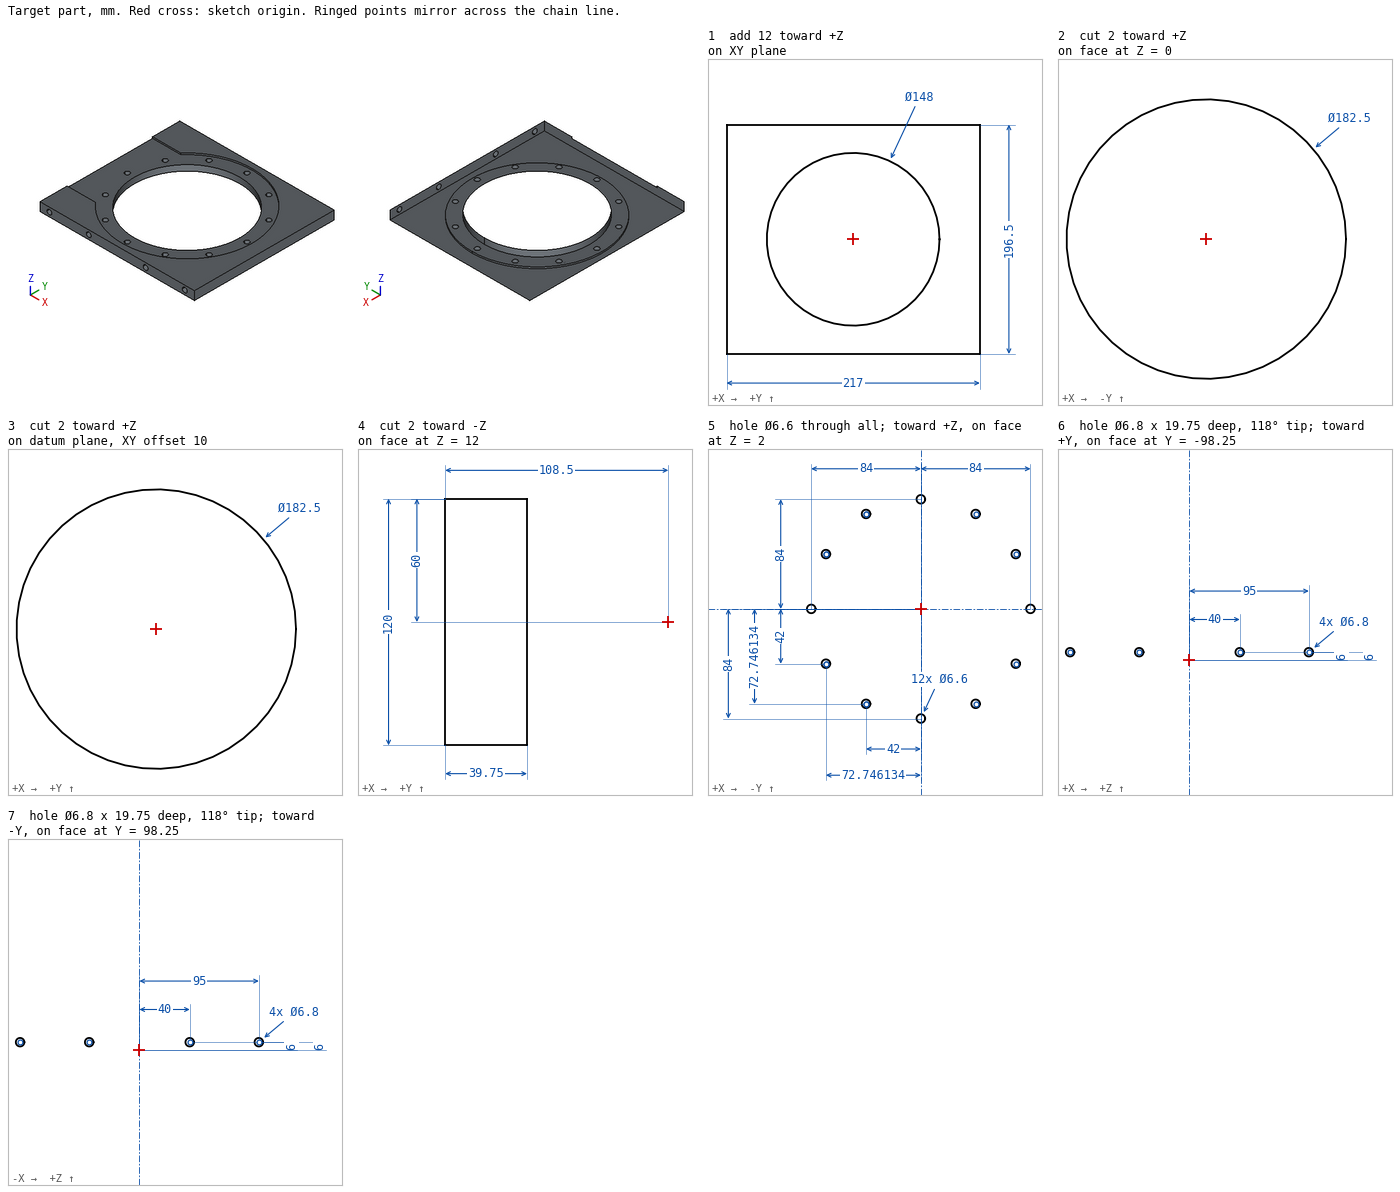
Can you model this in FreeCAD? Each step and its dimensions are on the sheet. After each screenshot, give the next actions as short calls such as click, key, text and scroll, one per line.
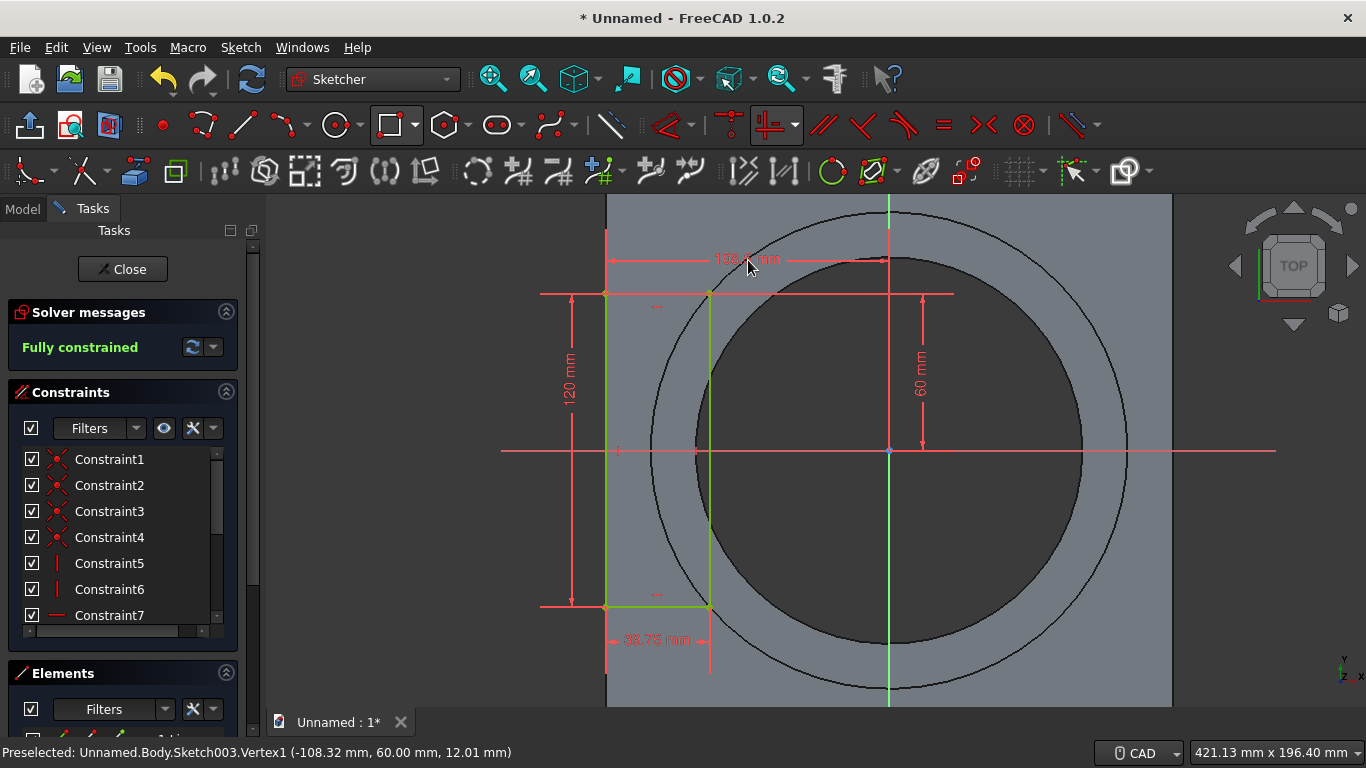
click(123, 269)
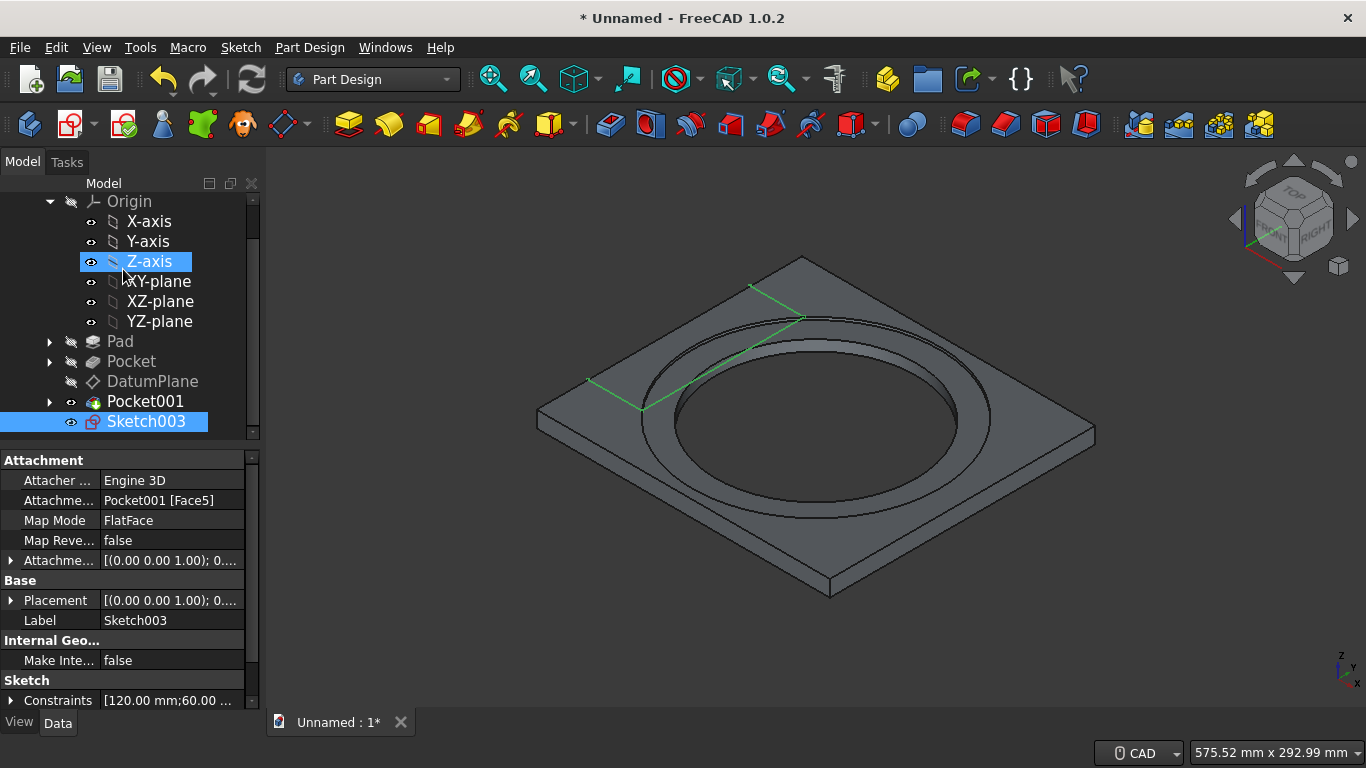
click(612, 124)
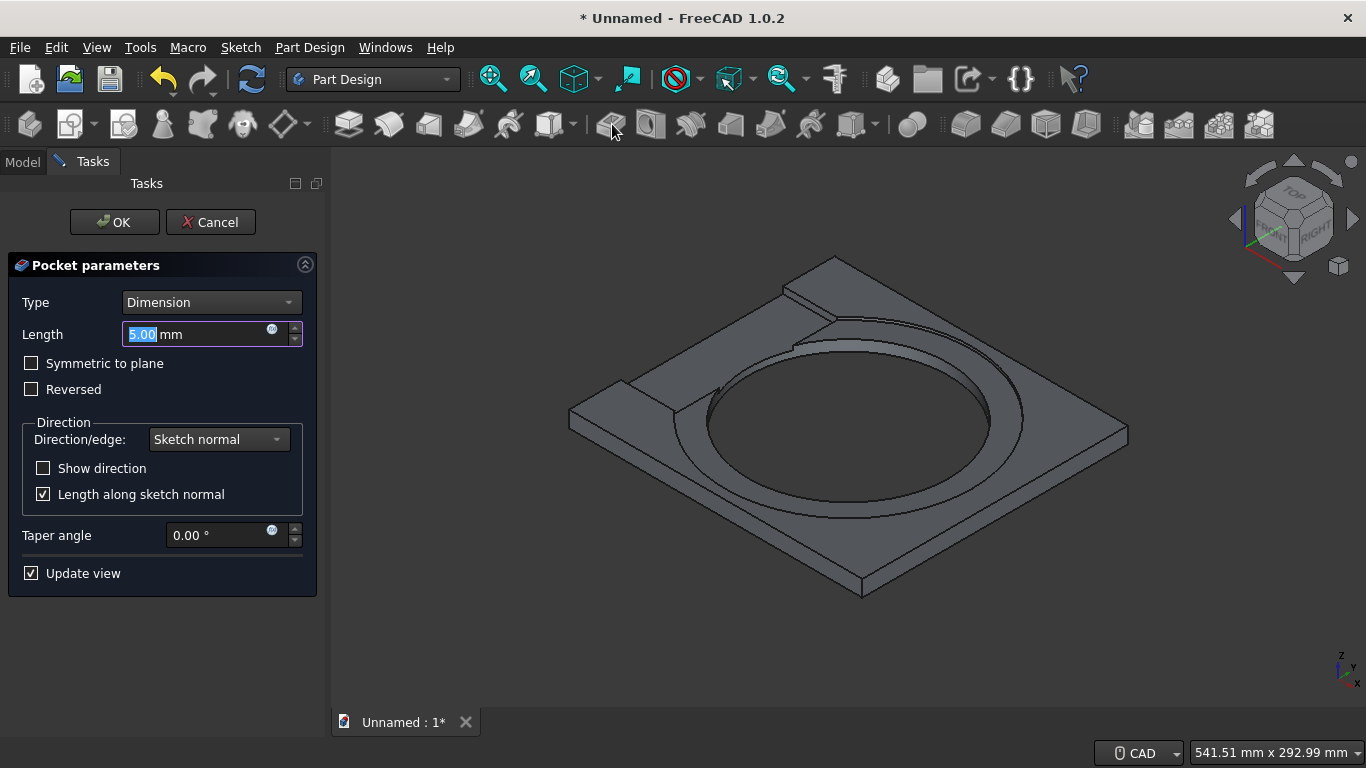
text(2)
key(Tab)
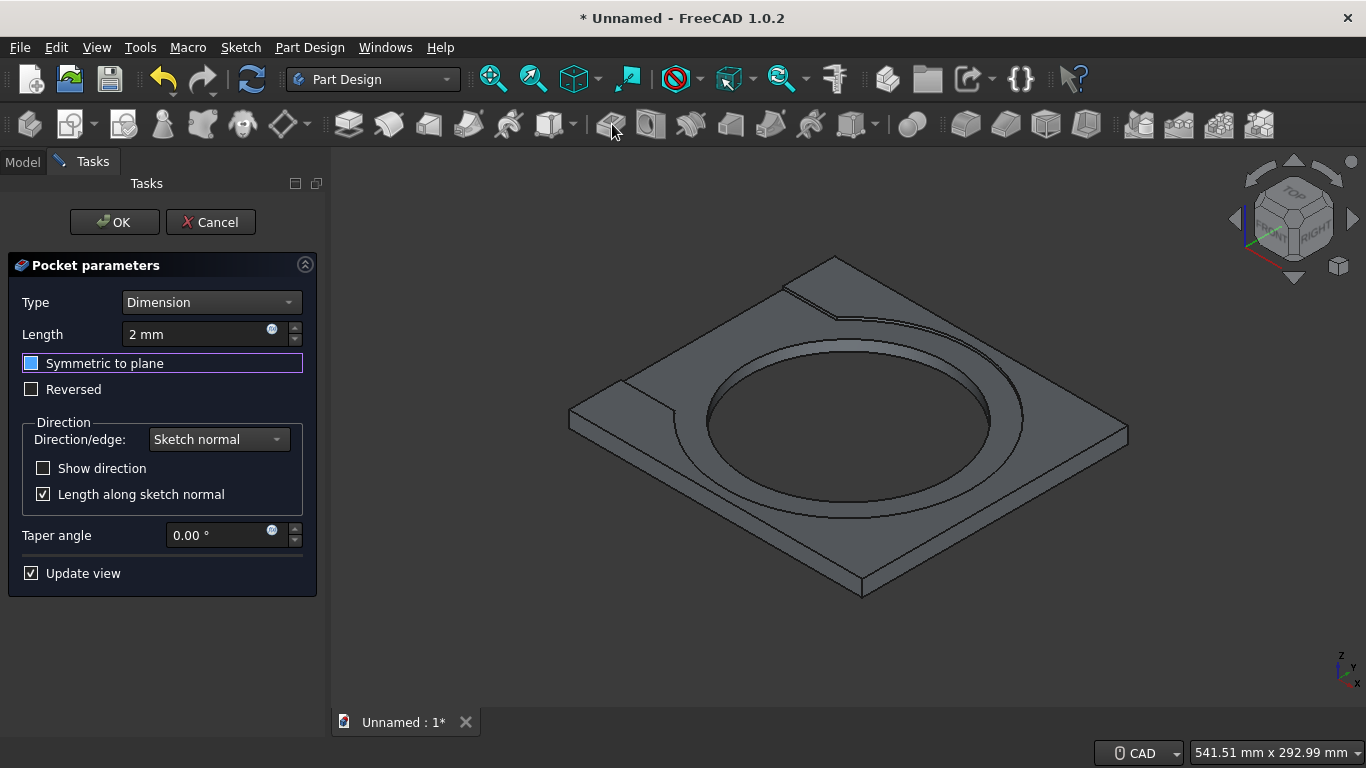
click(115, 222)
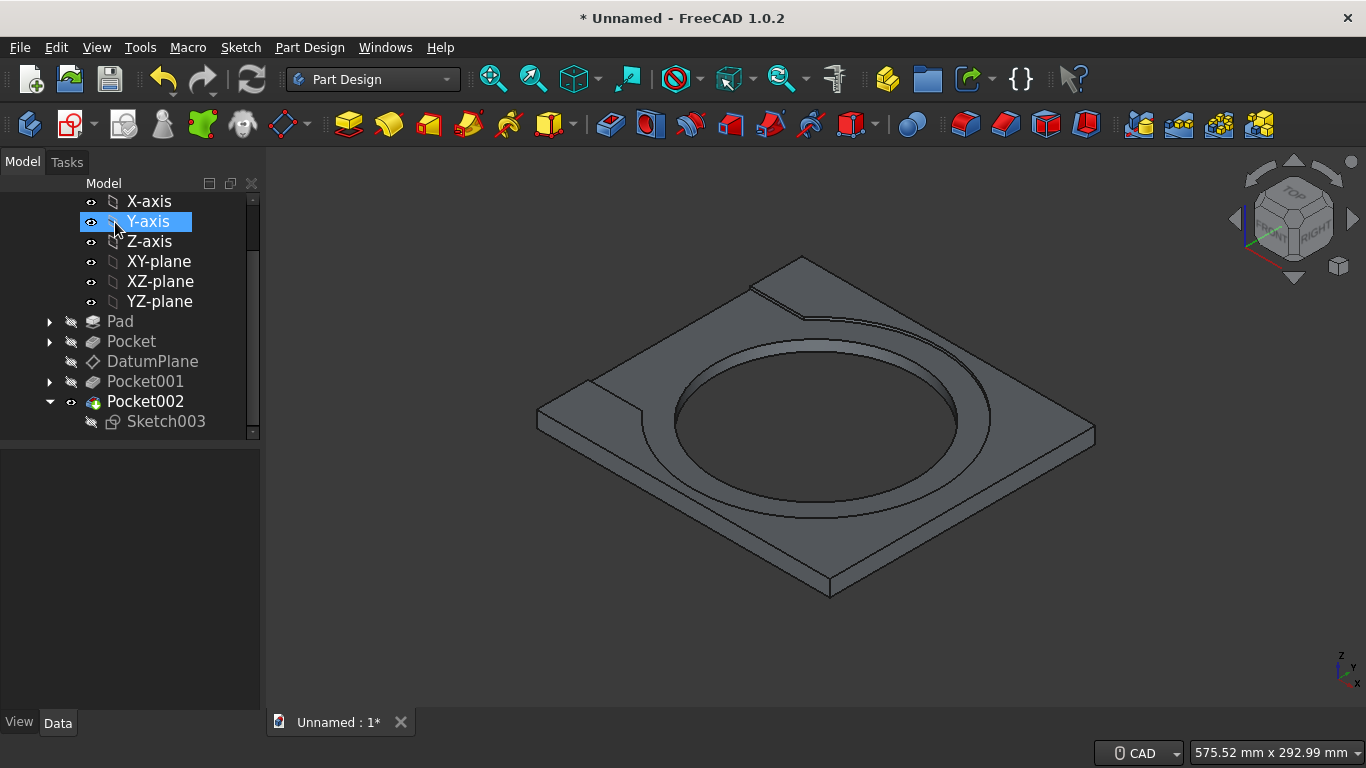
key(5)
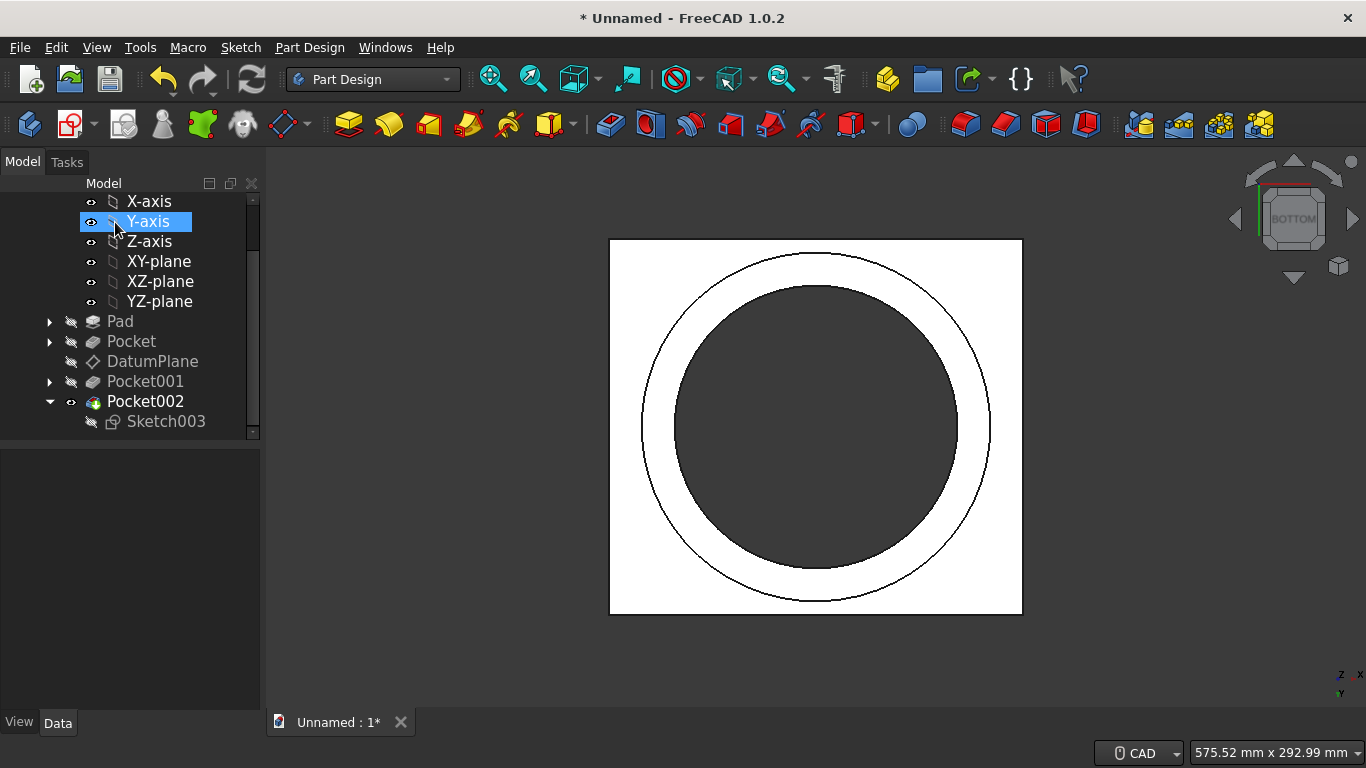
click(866, 575)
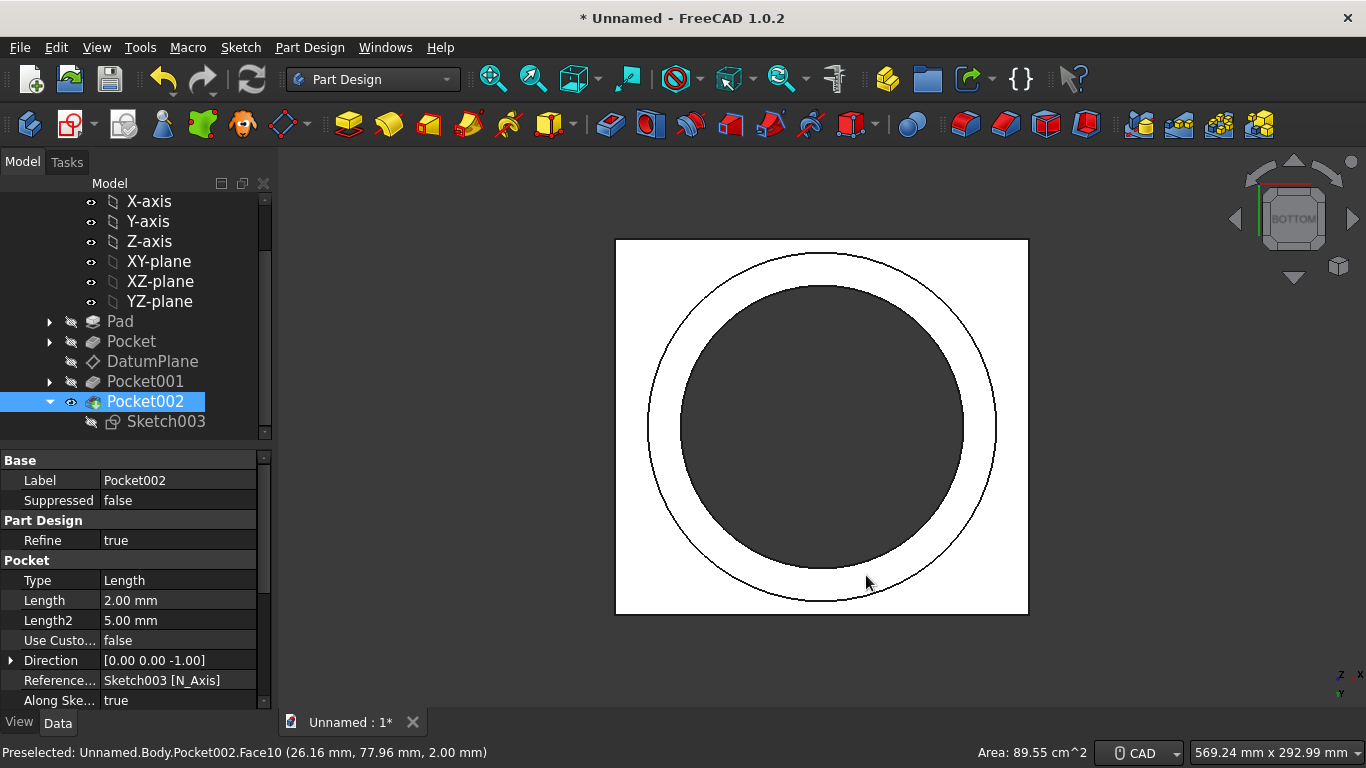
click(70, 124)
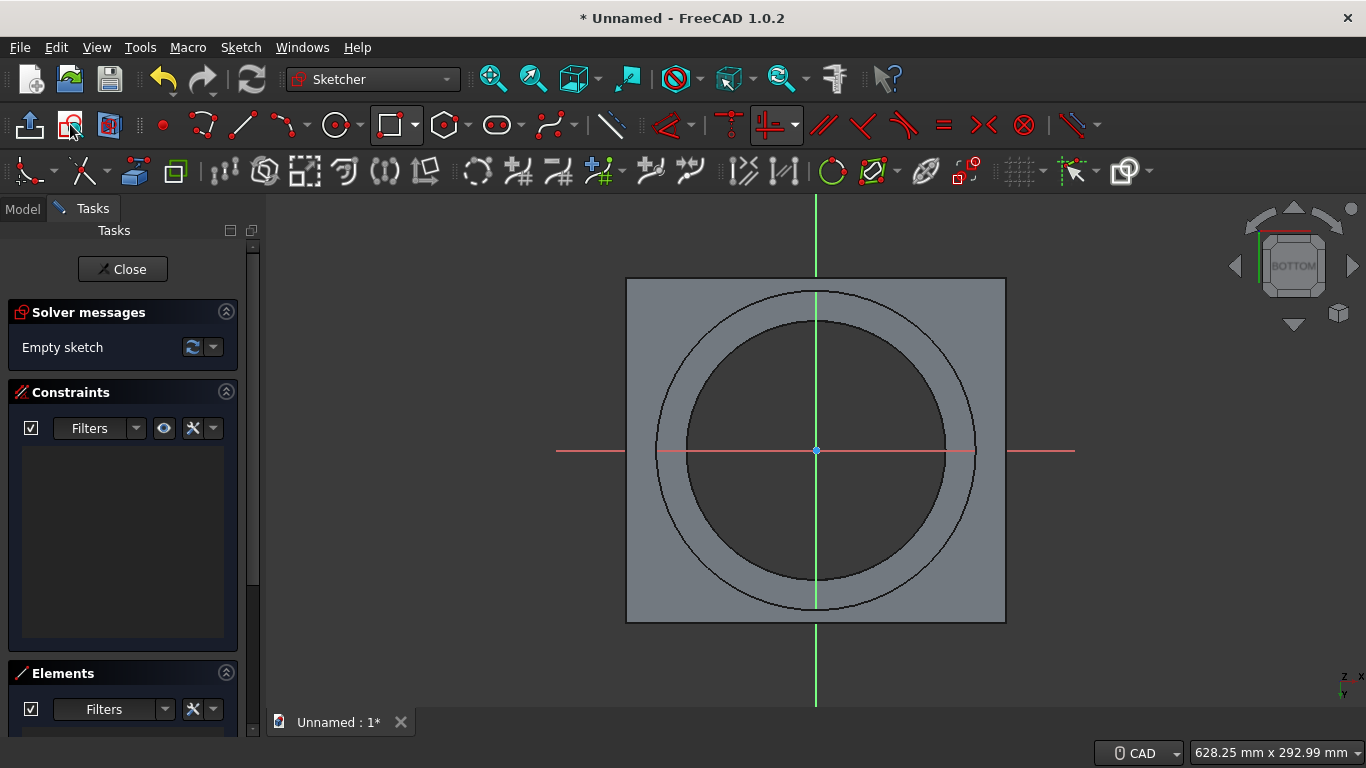
click(110, 126)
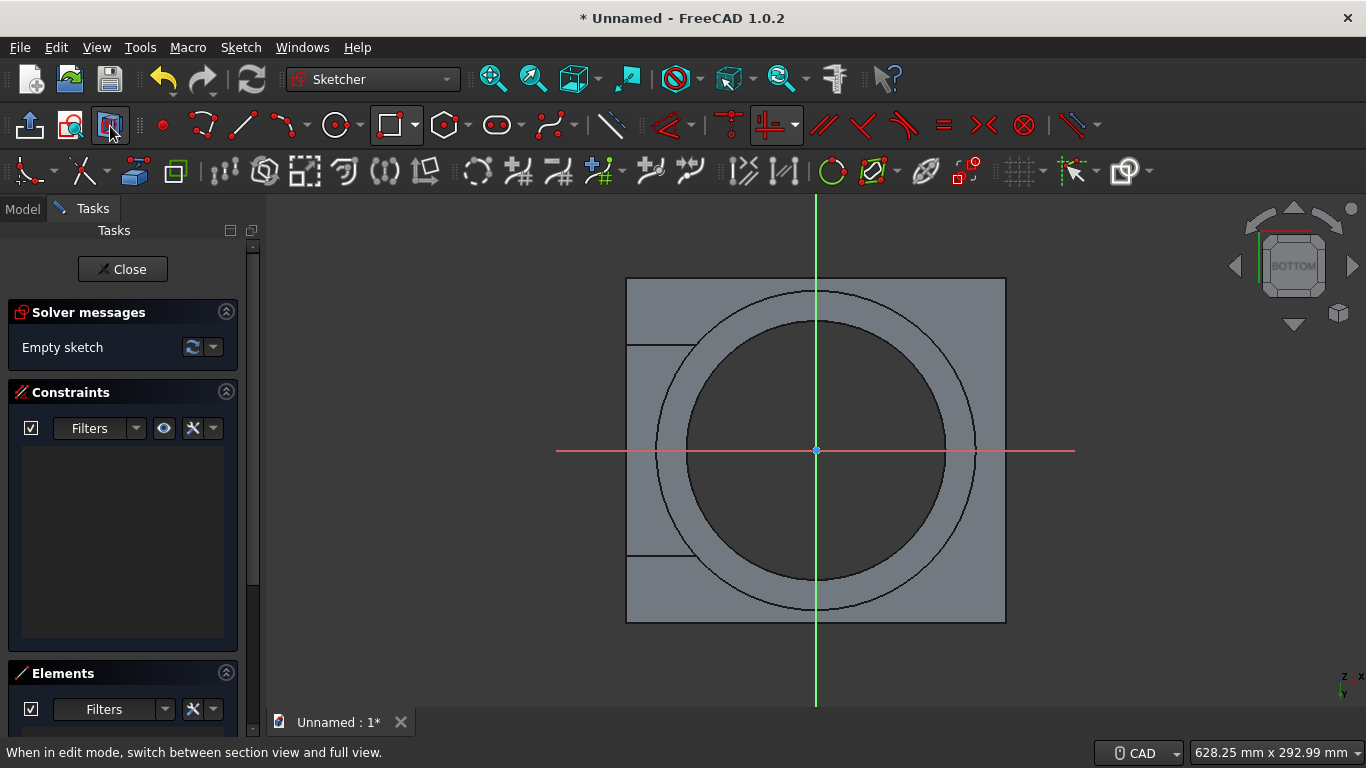
click(336, 126)